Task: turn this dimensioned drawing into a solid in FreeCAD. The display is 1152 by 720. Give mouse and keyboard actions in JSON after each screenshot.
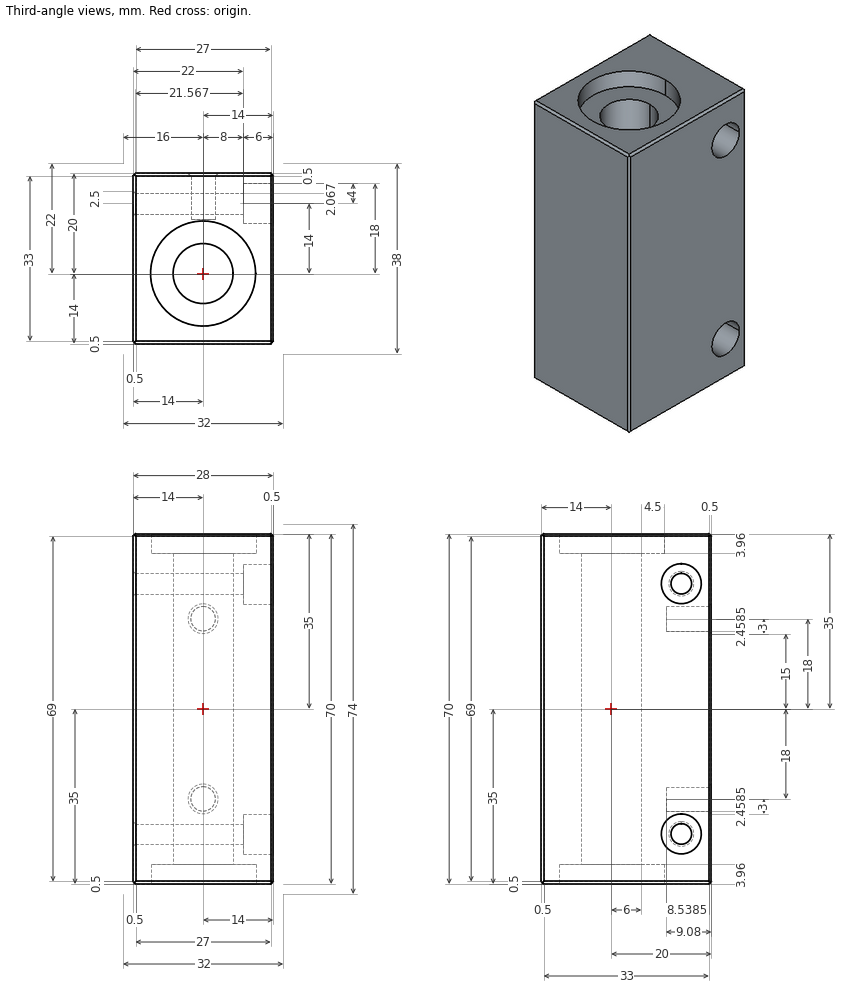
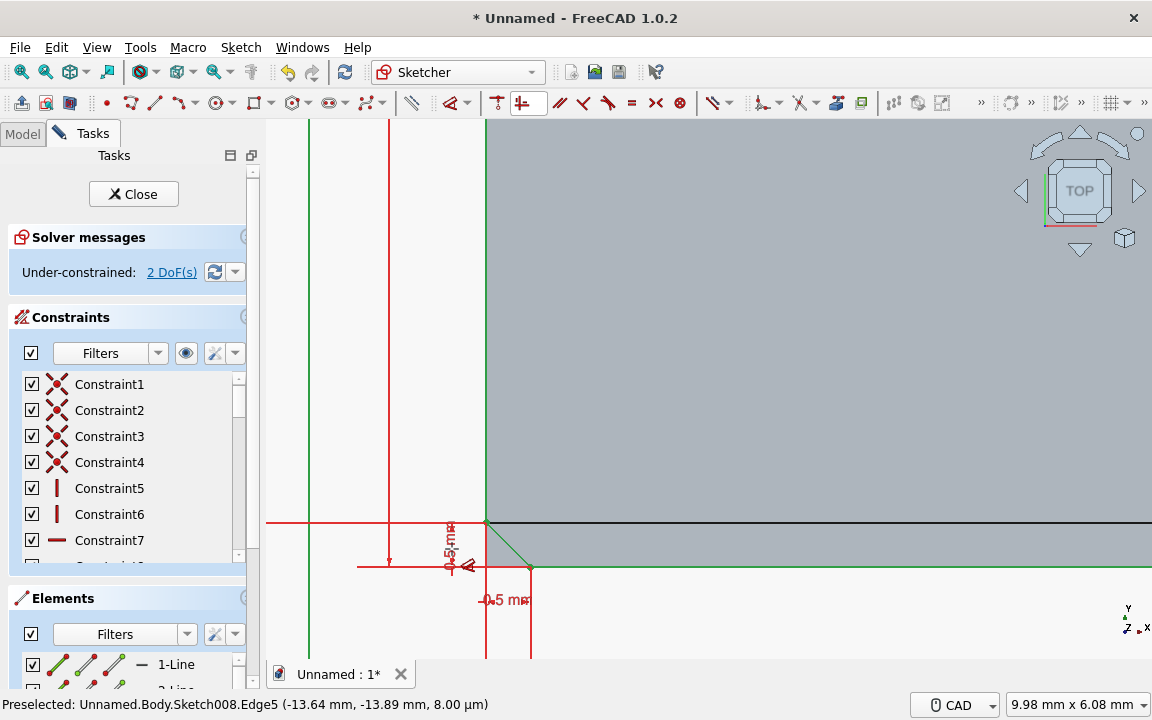
{"action": "scroll", "coordinate": [505, 555], "scroll_direction": "down", "scroll_amount": 11}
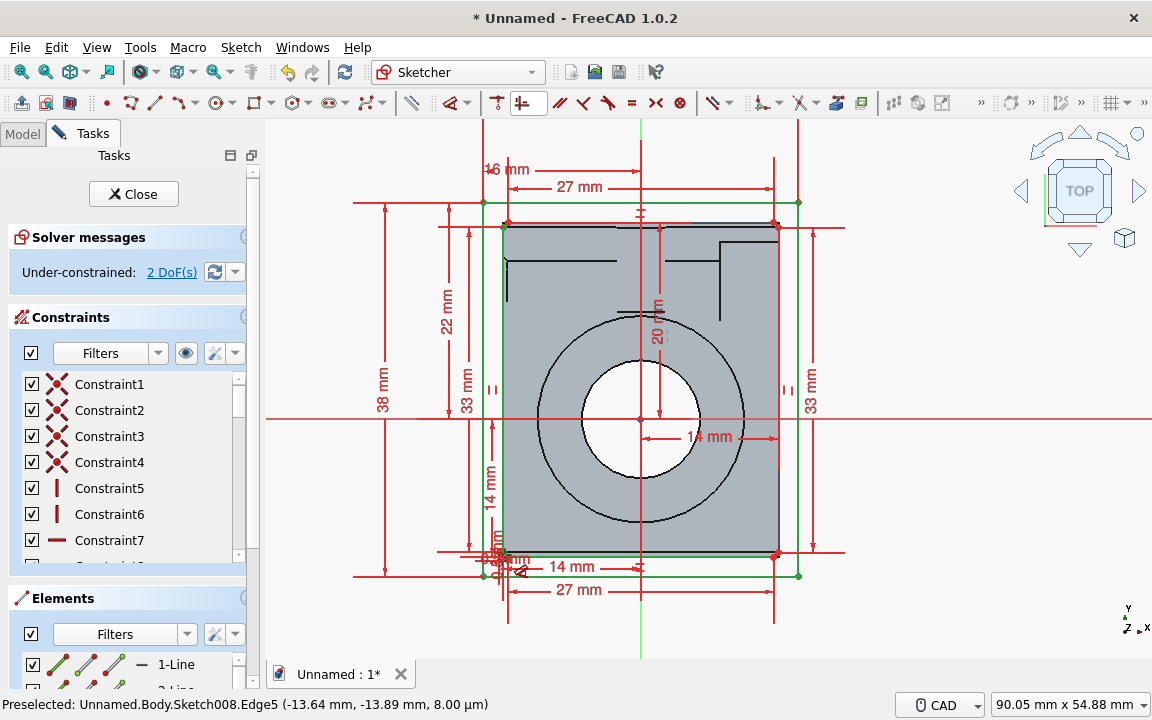
{"action": "scroll", "coordinate": [505, 226], "scroll_direction": "up", "scroll_amount": 11}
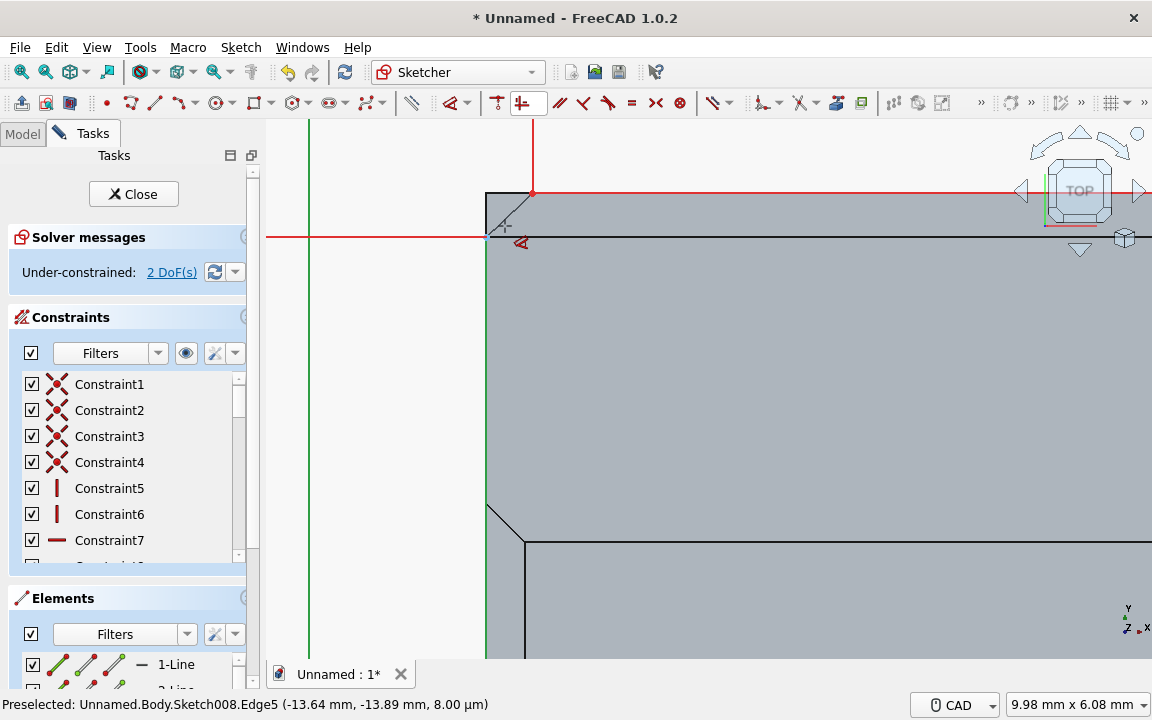
{"action": "left_click", "coordinate": [500, 224]}
{"action": "left_click", "coordinate": [510, 159]}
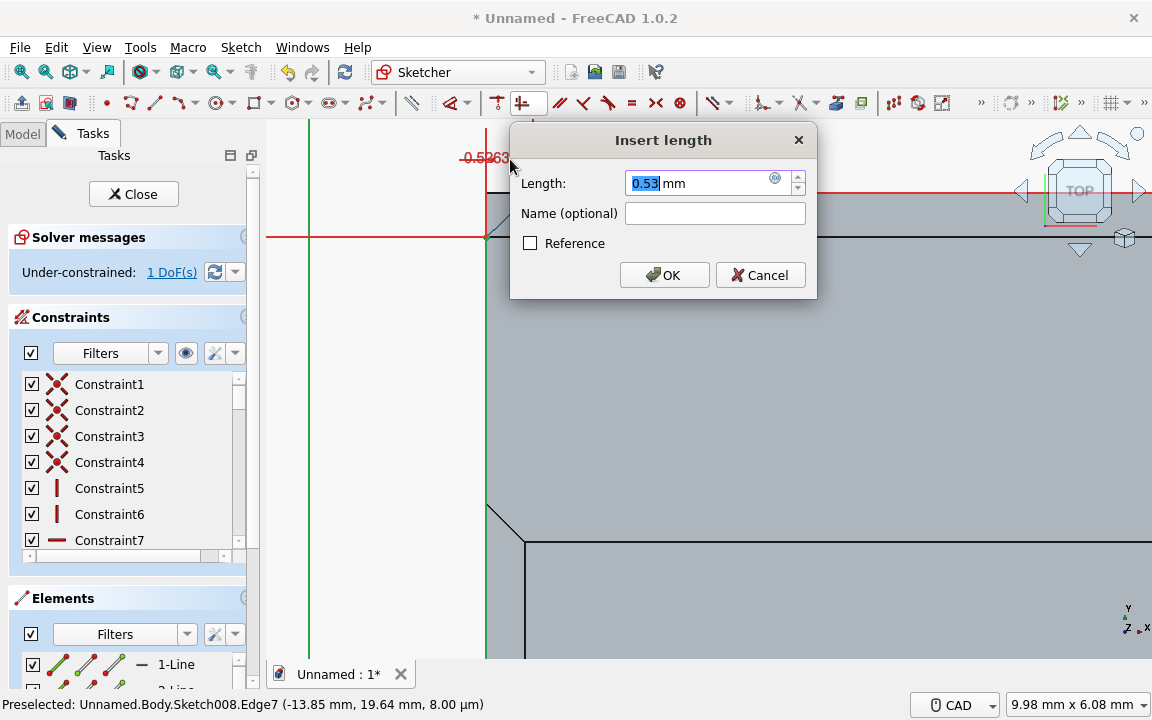
{"action": "type", "text": "0.5"}
{"action": "key", "text": "Return"}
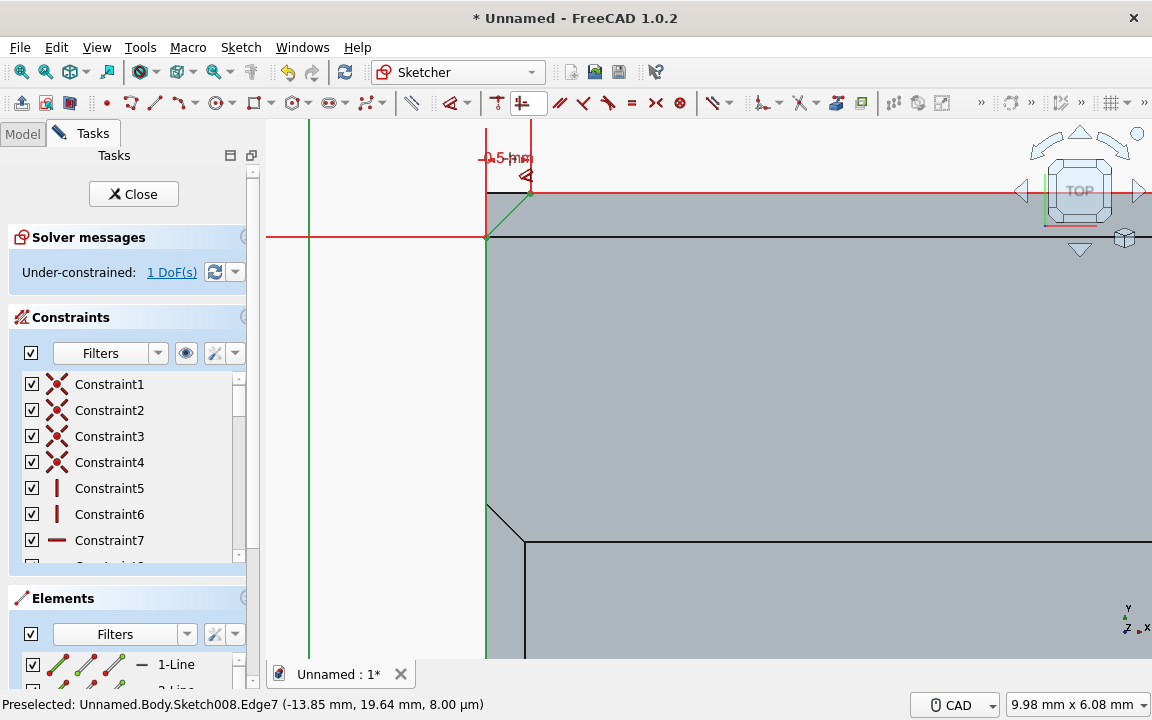
{"action": "scroll", "coordinate": [505, 225], "scroll_direction": "down", "scroll_amount": 11}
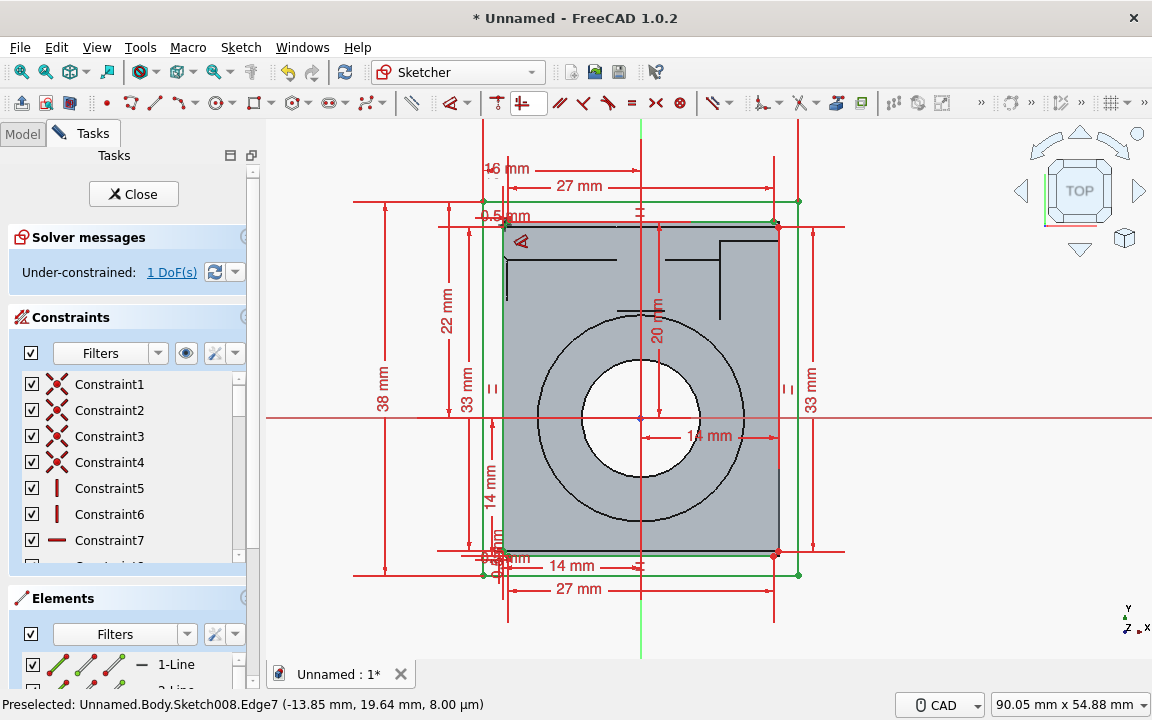
{"action": "scroll", "coordinate": [775, 223], "scroll_direction": "up", "scroll_amount": 11}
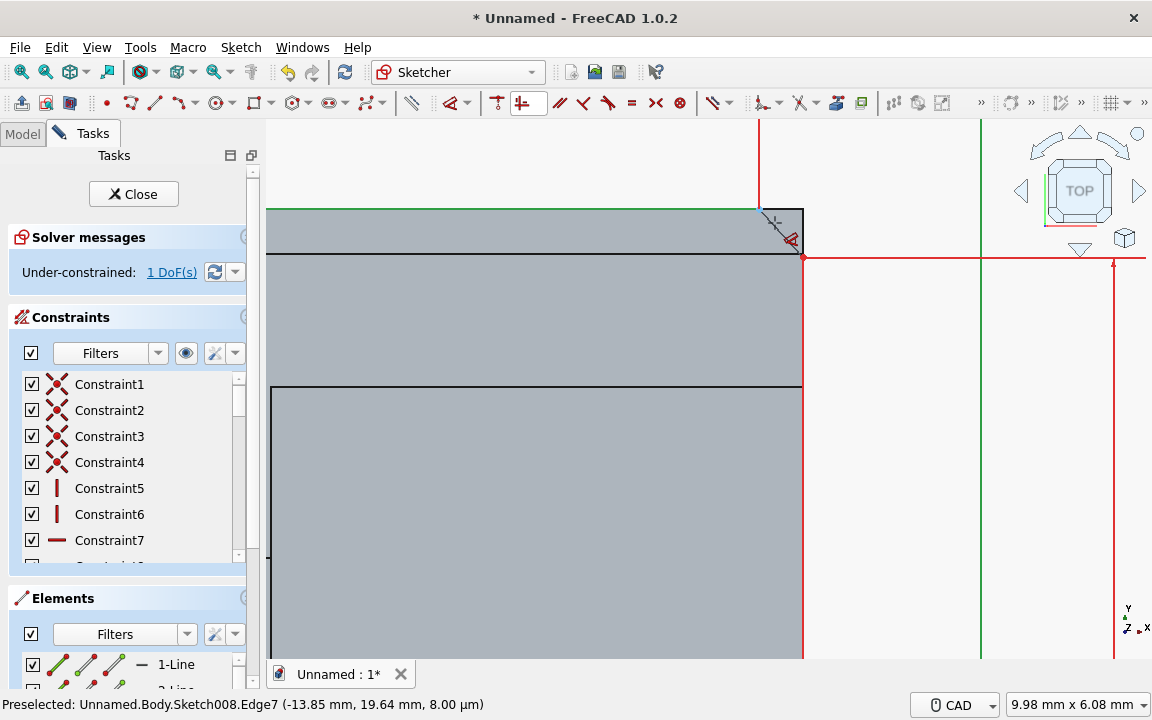
{"action": "left_click", "coordinate": [772, 224]}
{"action": "left_click", "coordinate": [837, 234]}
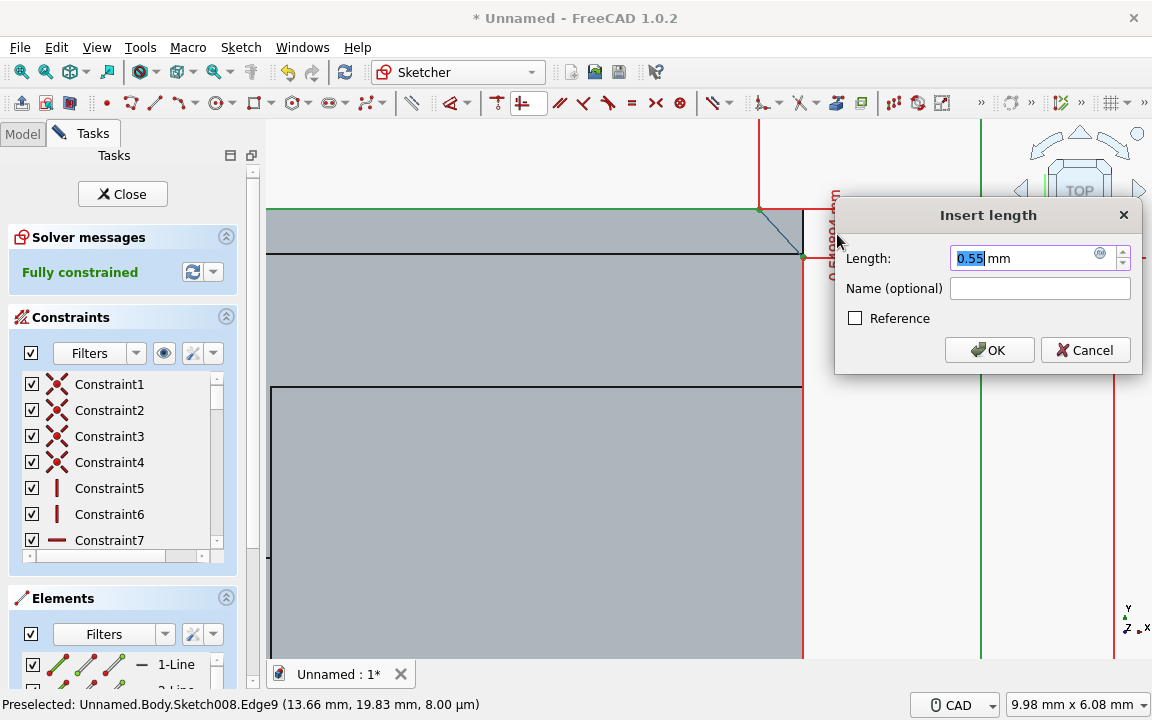
{"action": "type", "text": "0.5"}
{"action": "key", "text": "Return"}
{"action": "key", "text": "Escape"}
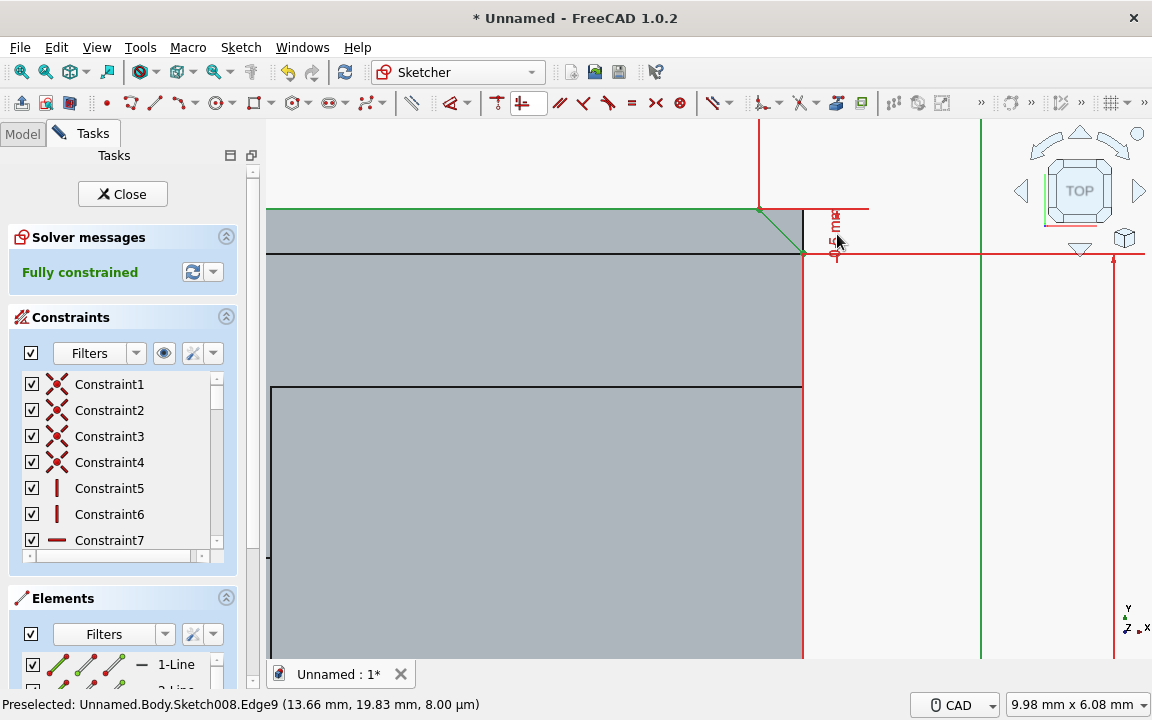
{"action": "left_click", "coordinate": [123, 194]}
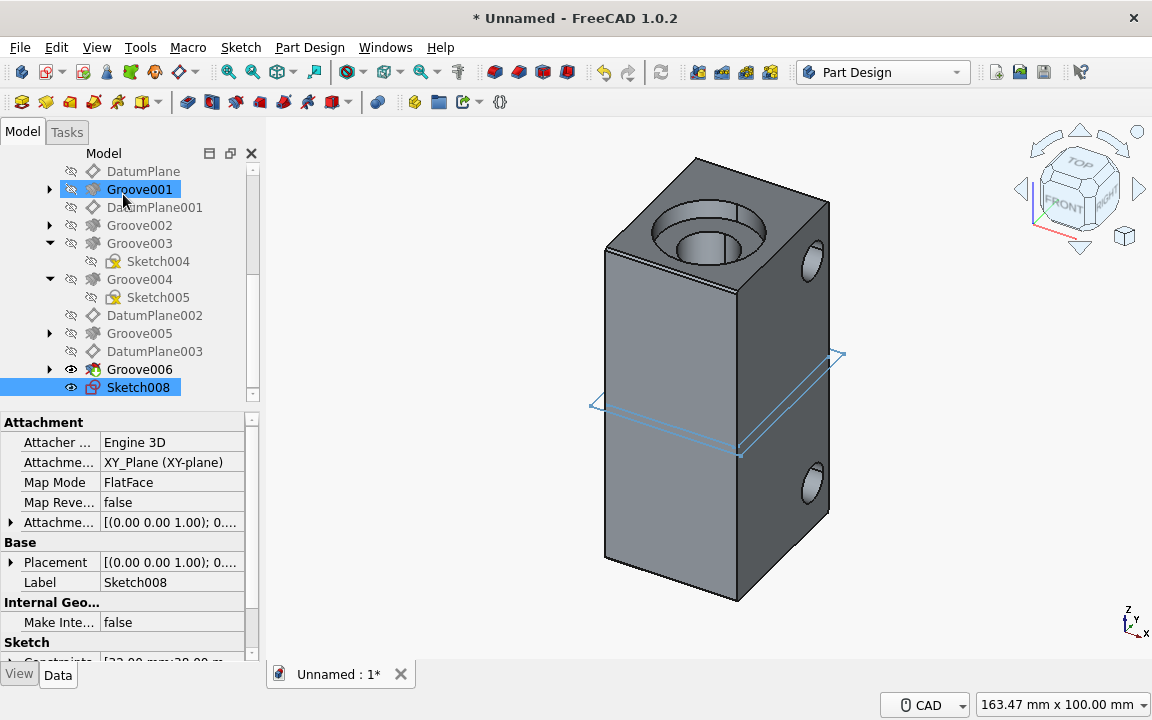
{"action": "left_click", "coordinate": [188, 102]}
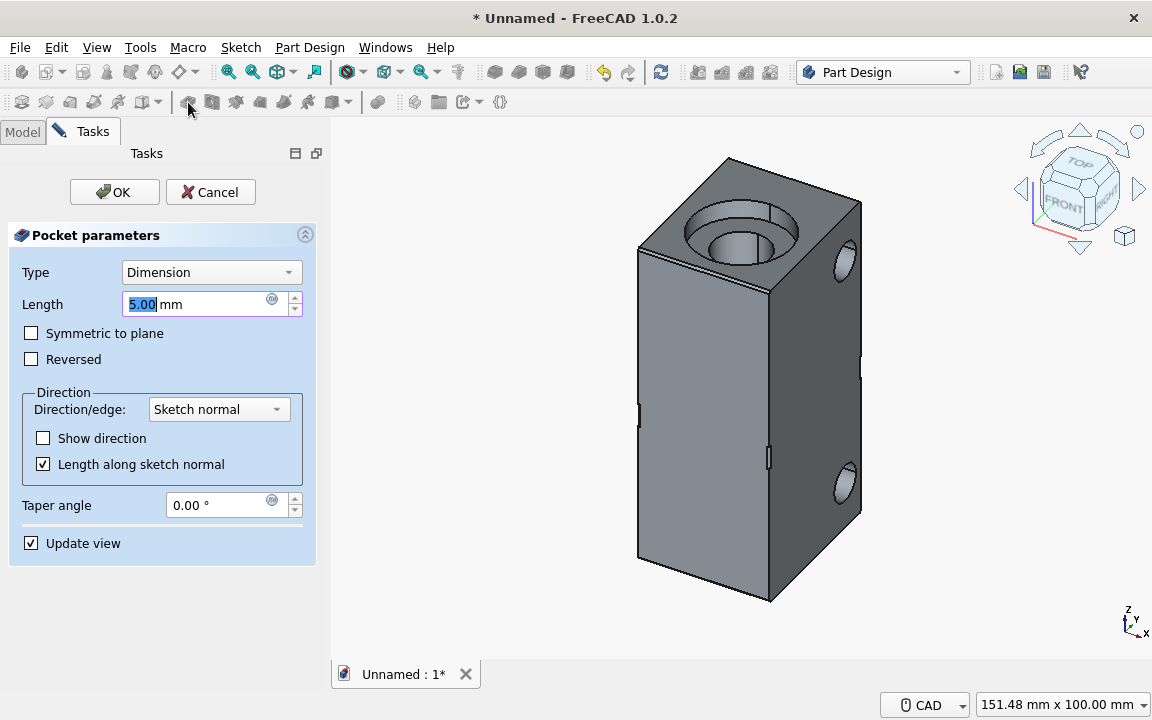
{"action": "type", "text": "70"}
{"action": "key", "text": "Tab"}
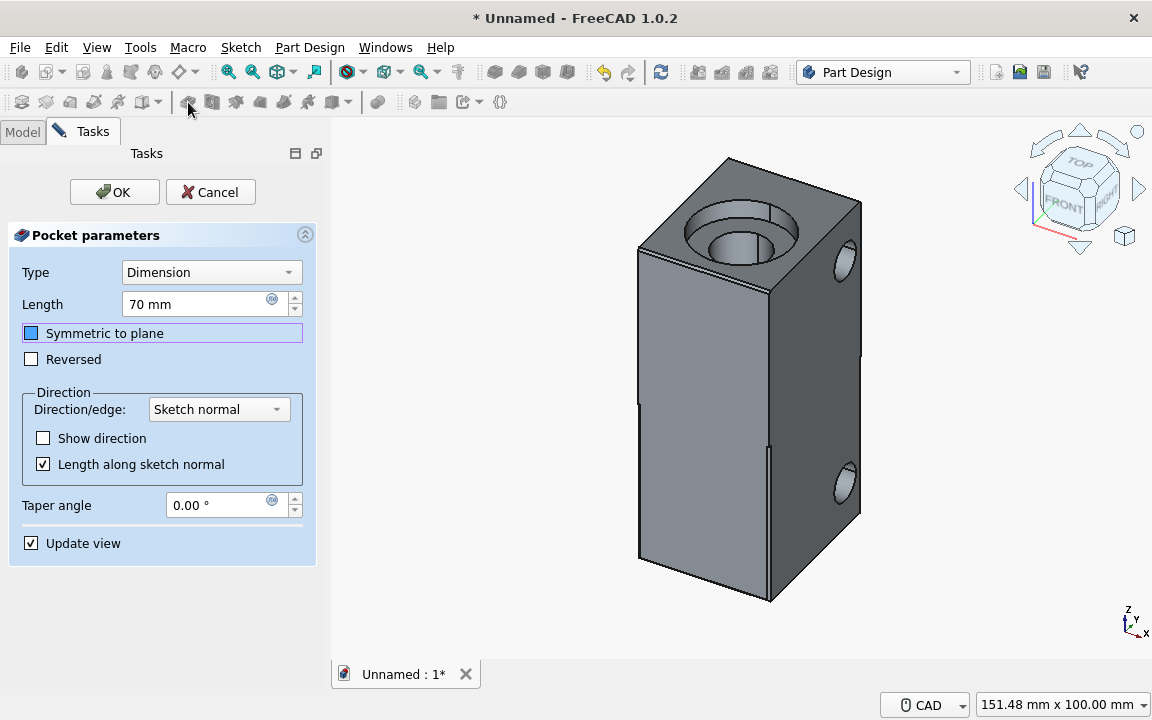
{"action": "left_click", "coordinate": [30, 333]}